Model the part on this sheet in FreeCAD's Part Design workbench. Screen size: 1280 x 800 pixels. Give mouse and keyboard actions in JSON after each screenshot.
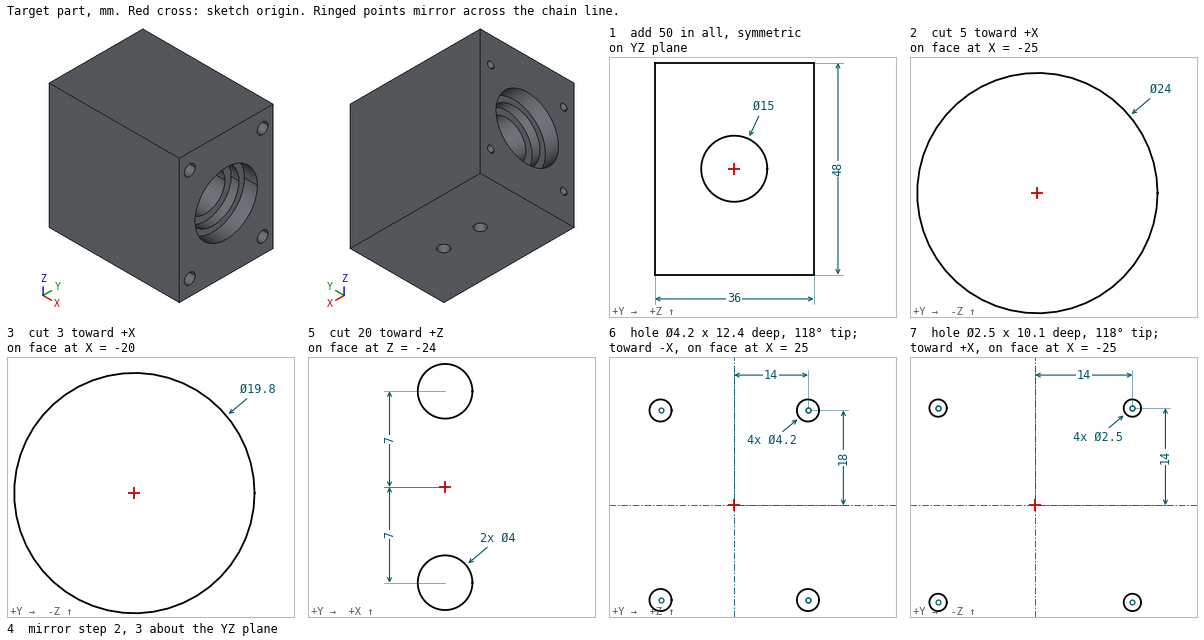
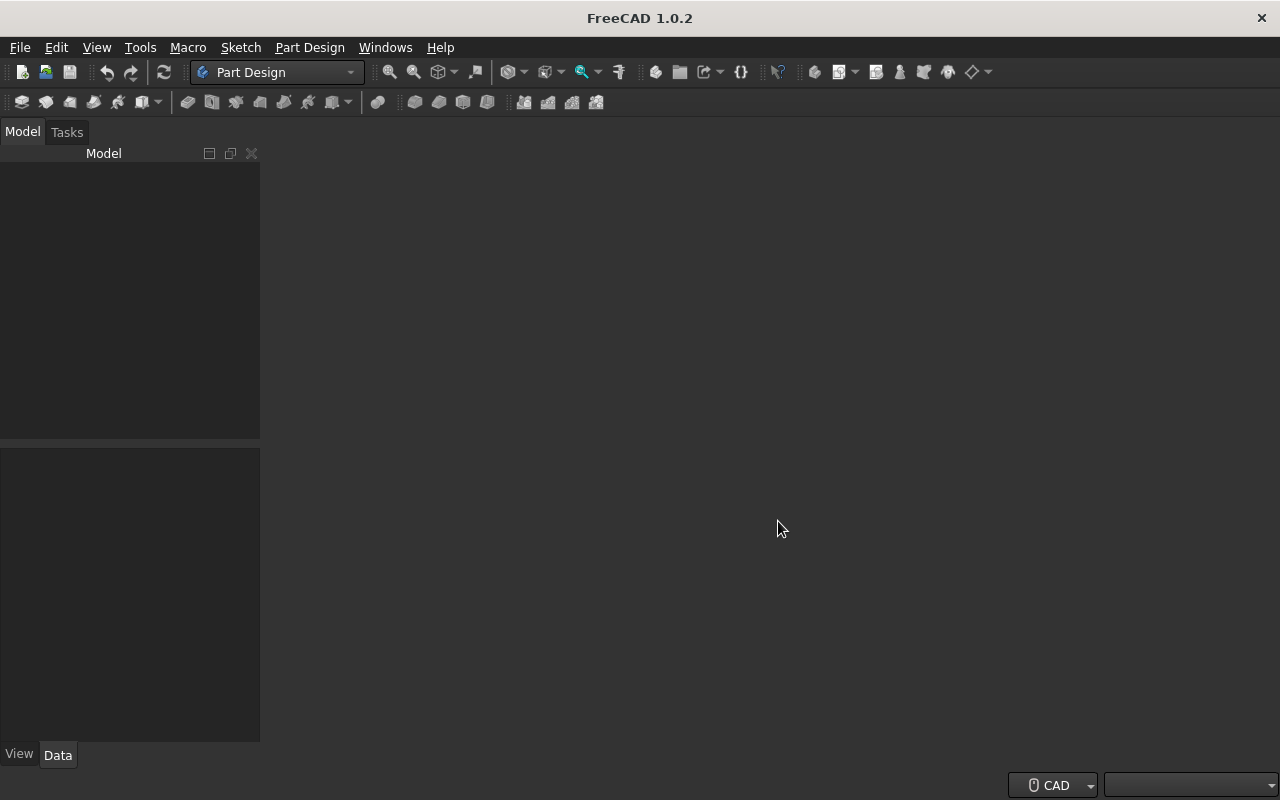
{"action": "left_click", "coordinate": [22, 72]}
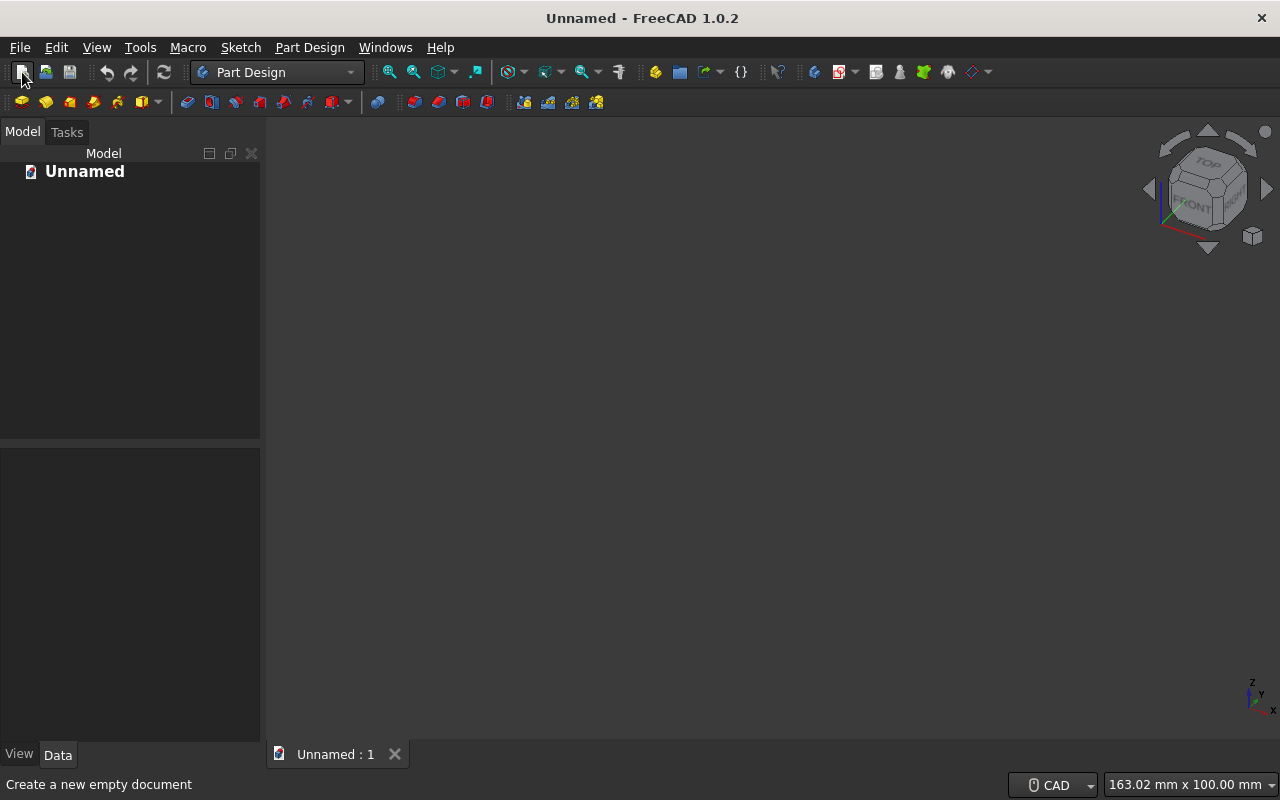
{"action": "left_click", "coordinate": [840, 72]}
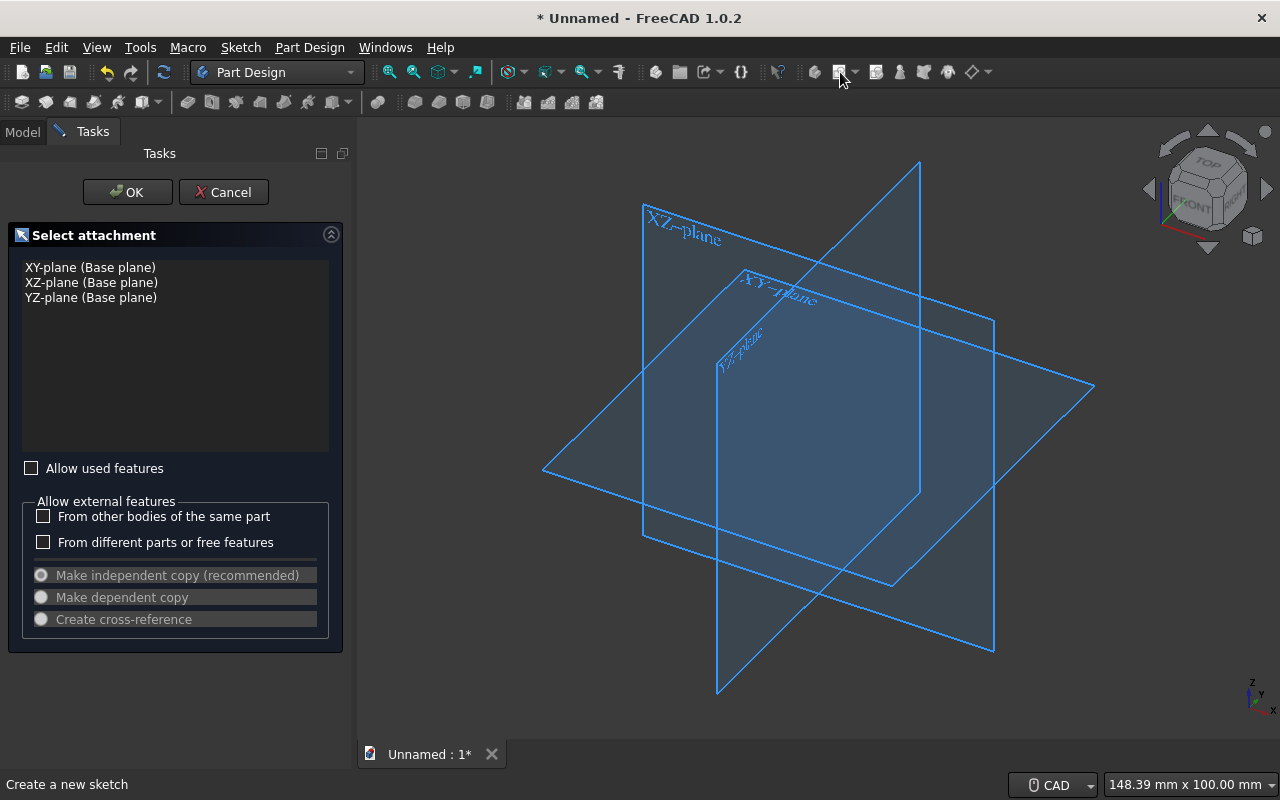
{"action": "left_click", "coordinate": [82, 298]}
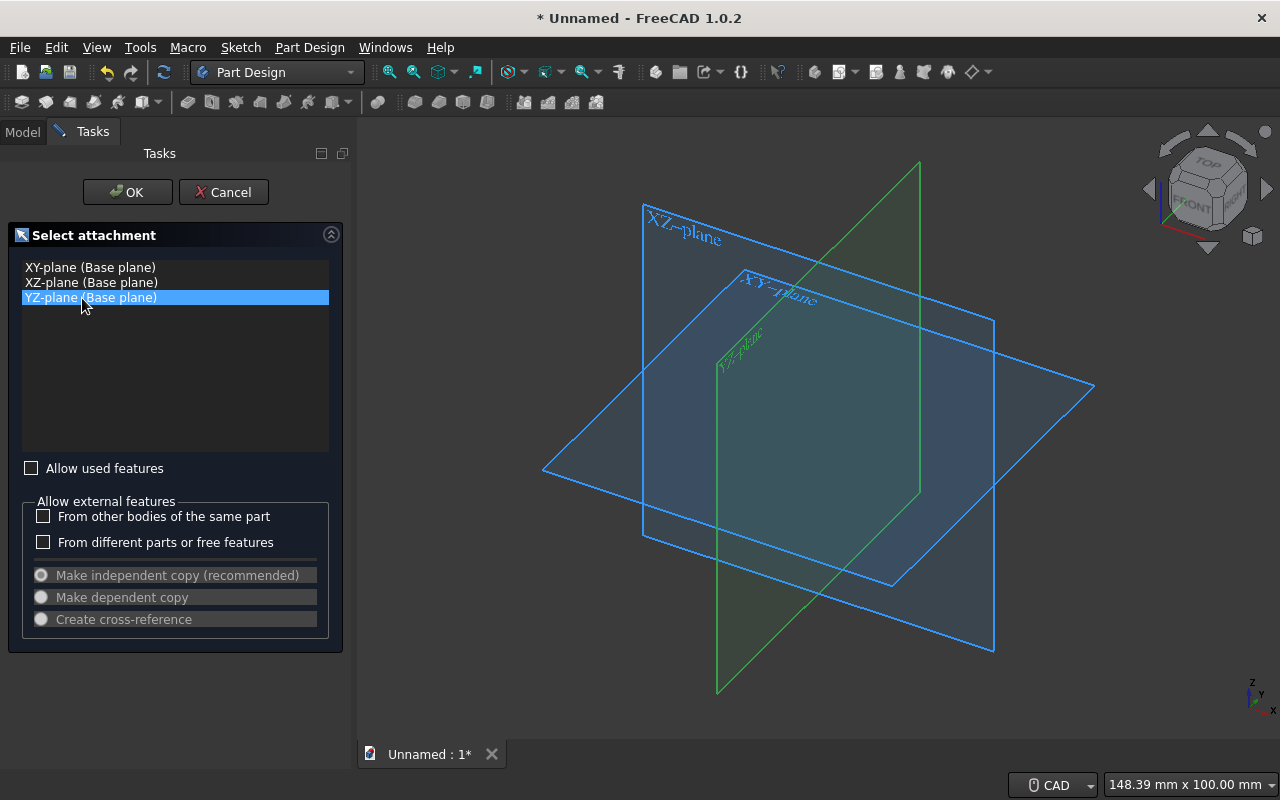
{"action": "left_click", "coordinate": [128, 192]}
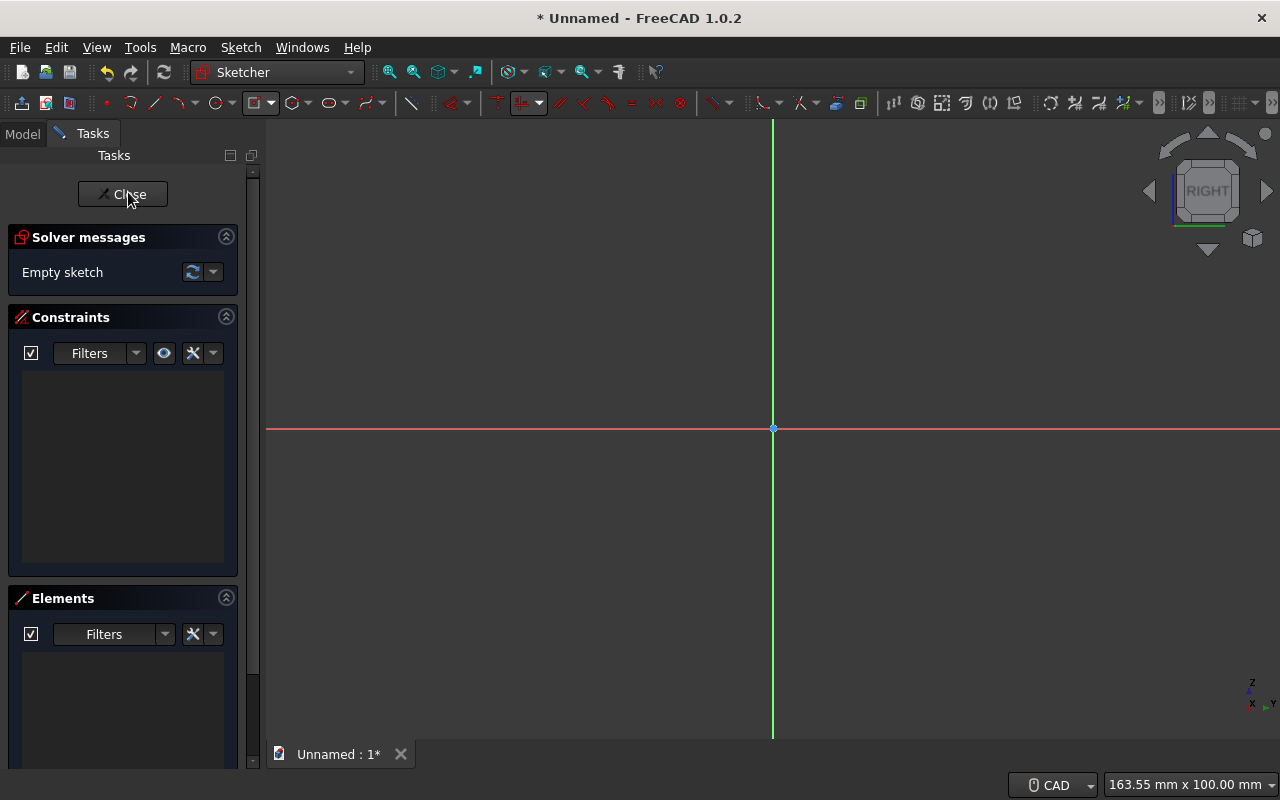
{"action": "left_click", "coordinate": [254, 104]}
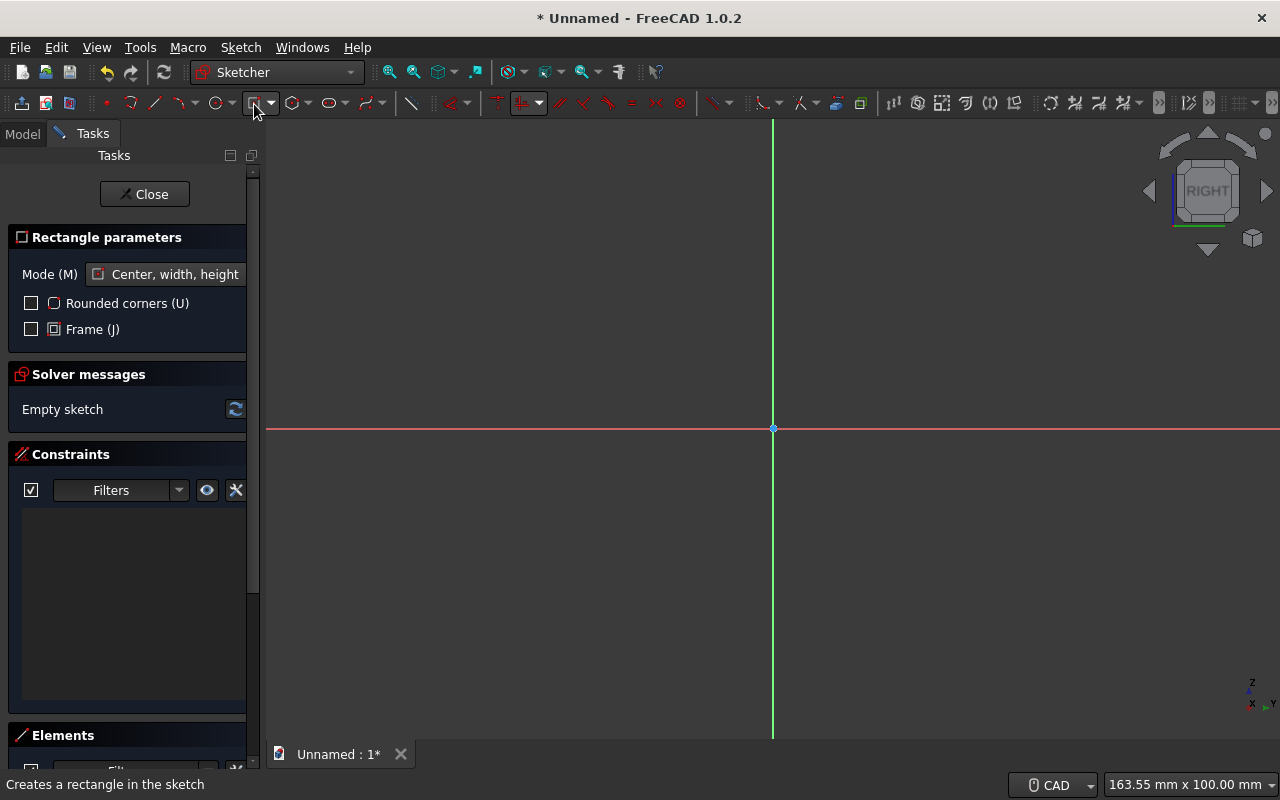
{"action": "left_click", "coordinate": [773, 429]}
{"action": "left_click", "coordinate": [885, 280]}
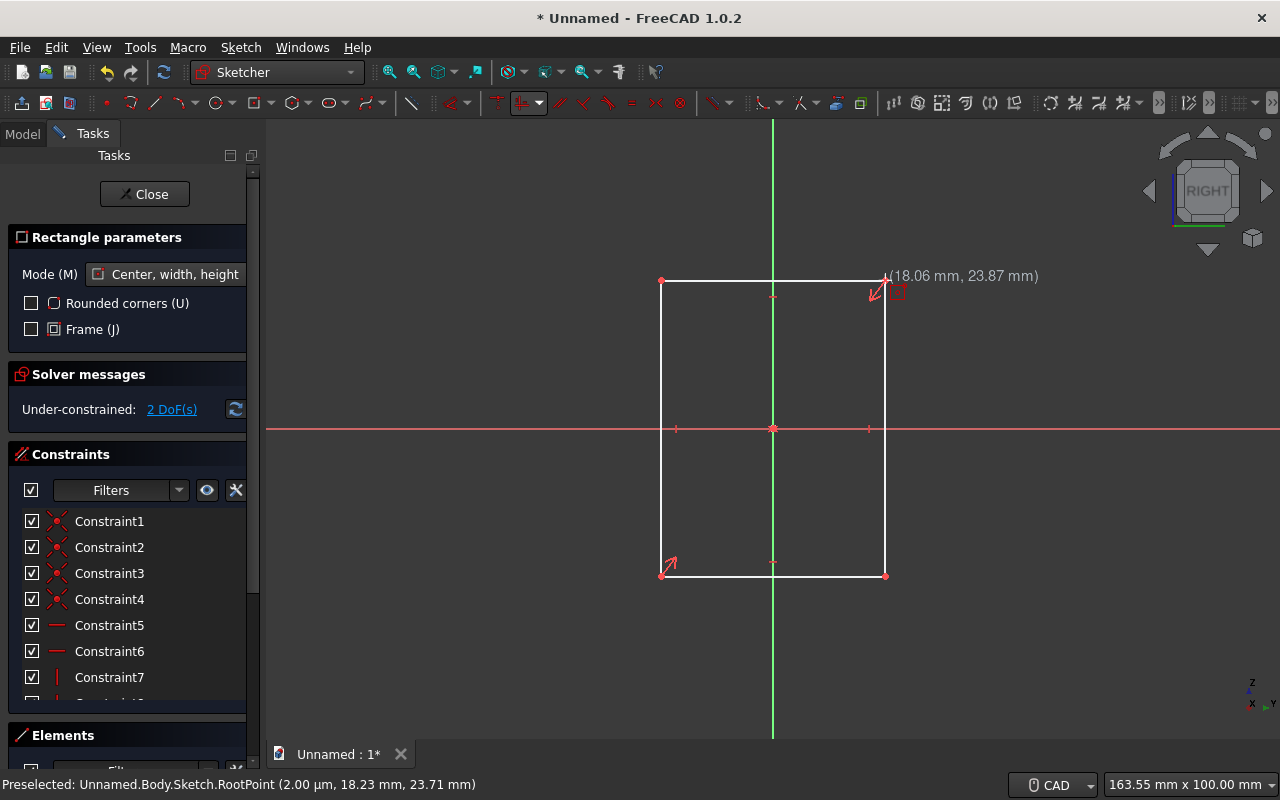
{"action": "left_click", "coordinate": [216, 104]}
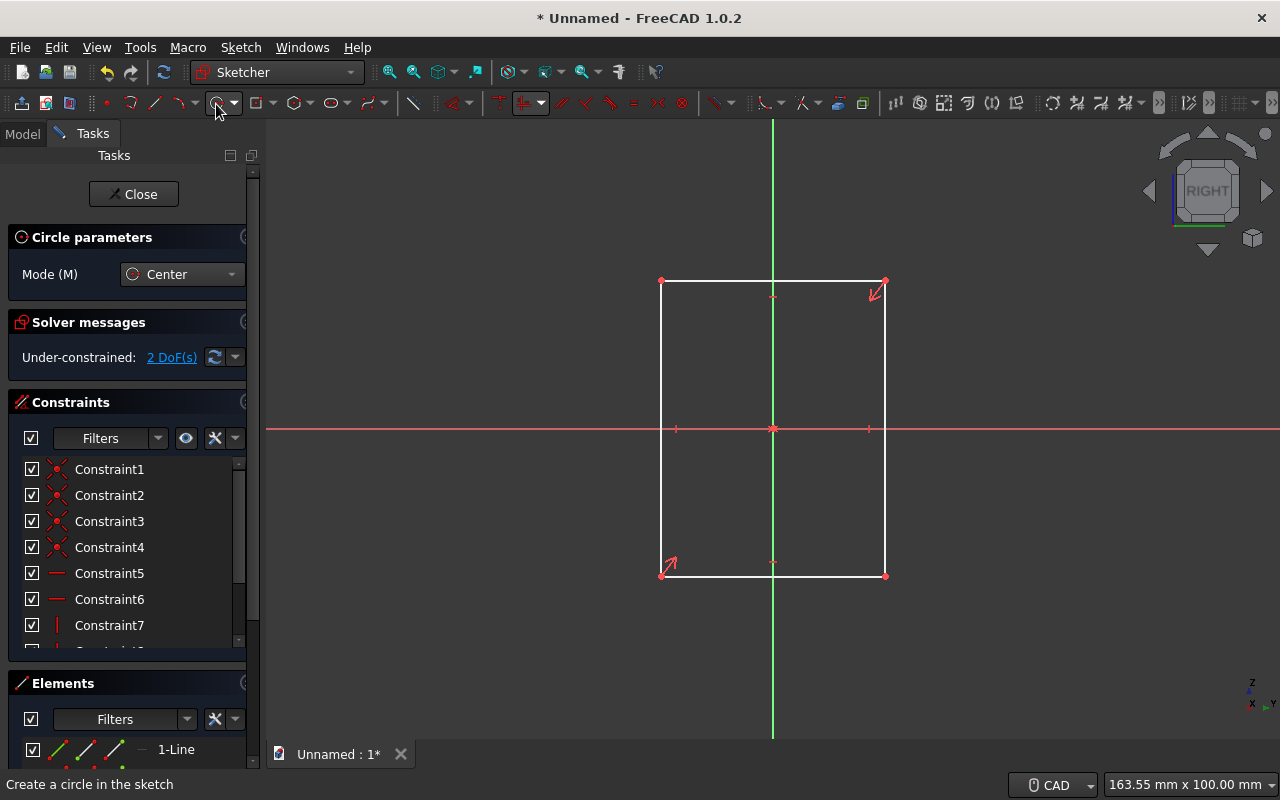
{"action": "left_click", "coordinate": [773, 429]}
{"action": "left_click", "coordinate": [806, 396]}
{"action": "key", "text": "Escape"}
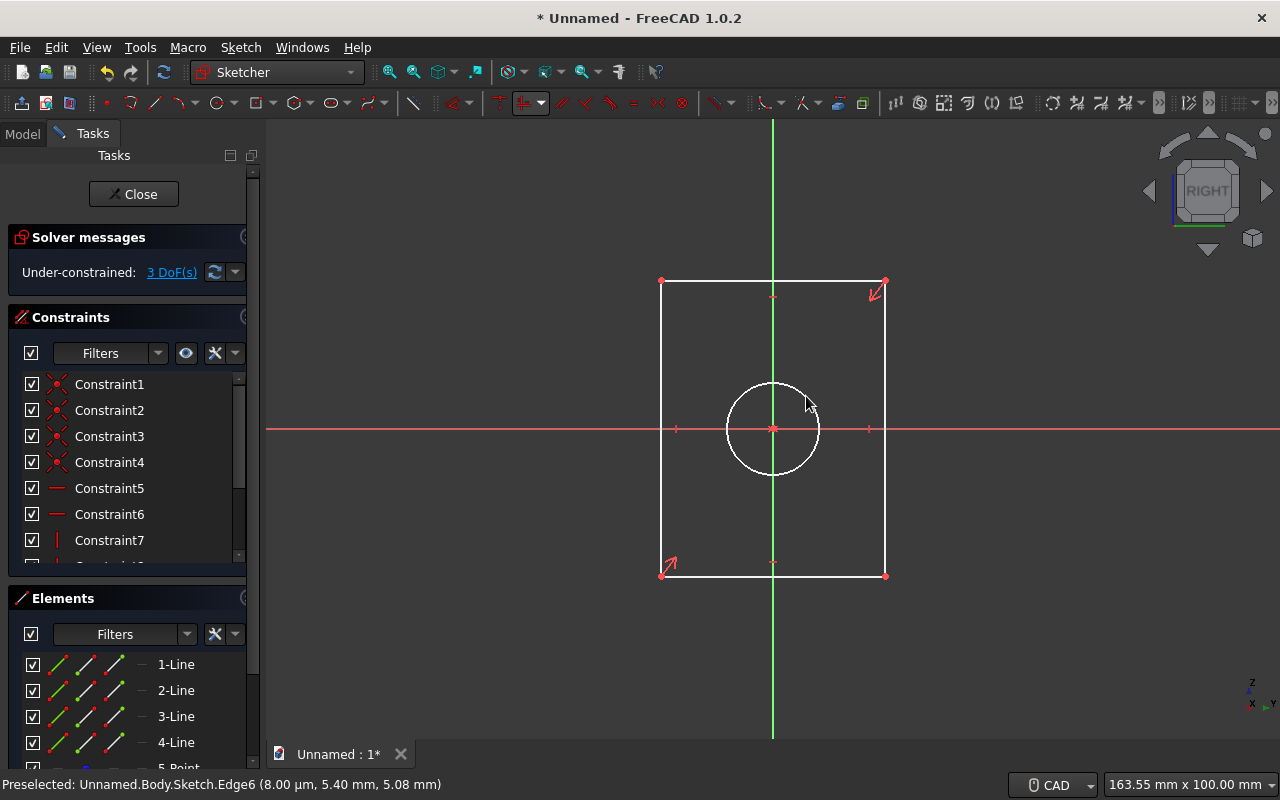
{"action": "left_click", "coordinate": [805, 396]}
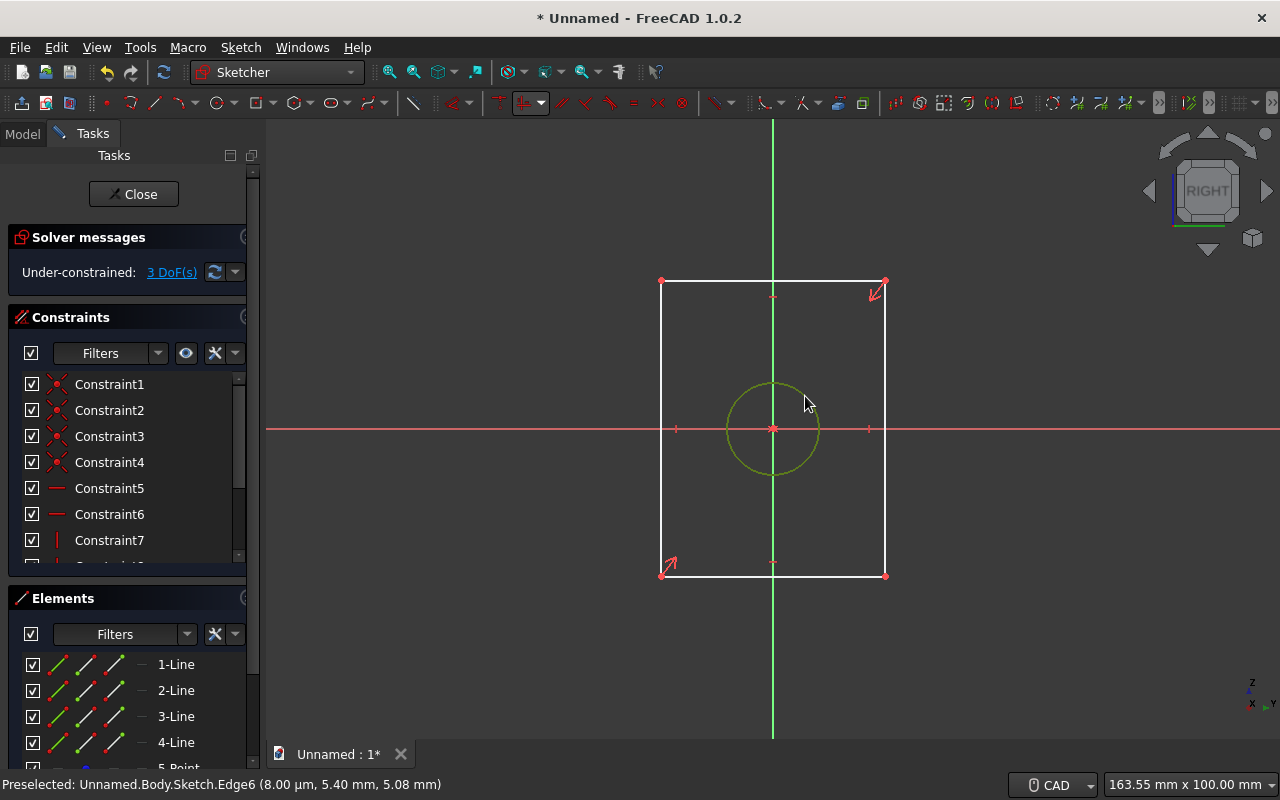
{"action": "left_click", "coordinate": [472, 104]}